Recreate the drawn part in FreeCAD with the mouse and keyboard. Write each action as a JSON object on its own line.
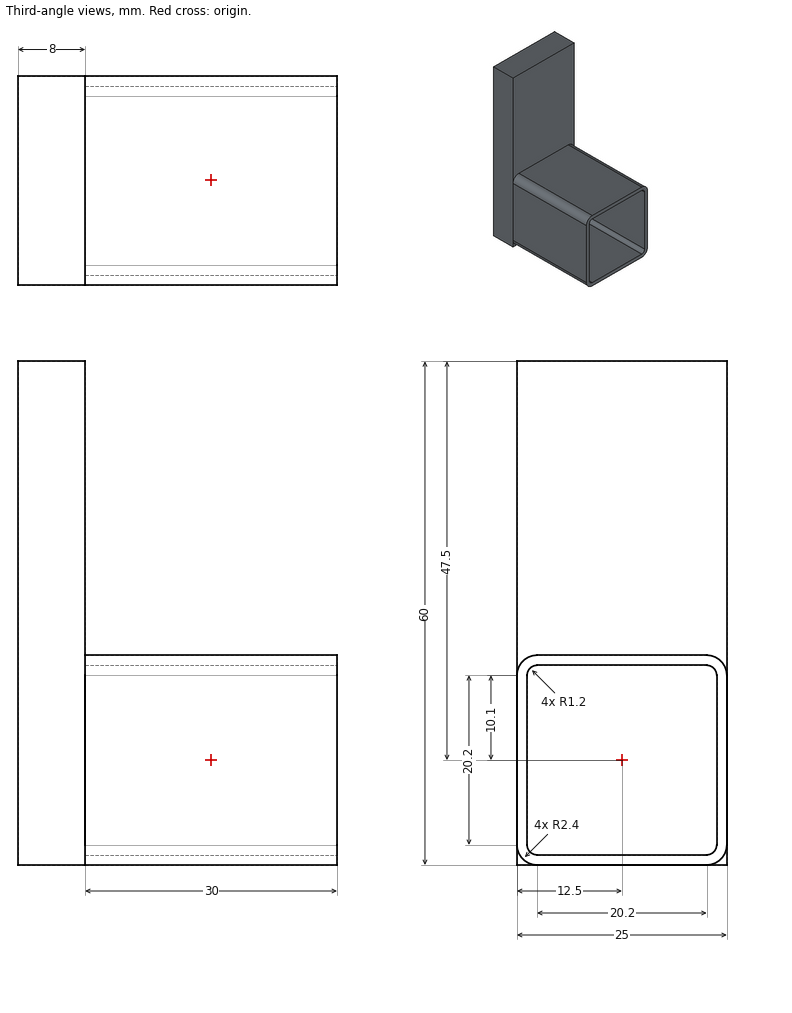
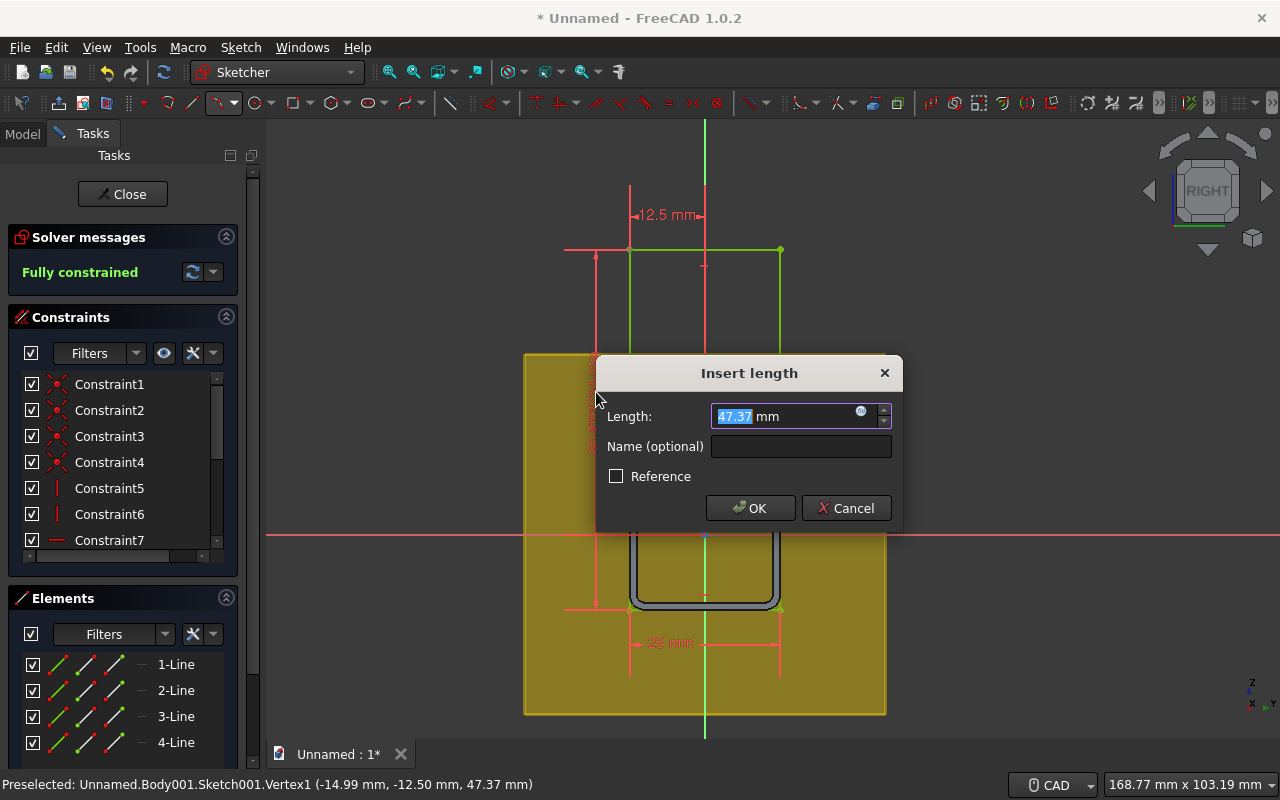
{"action": "type", "text": "47.5"}
{"action": "key", "text": "Return"}
{"action": "key", "text": "Escape"}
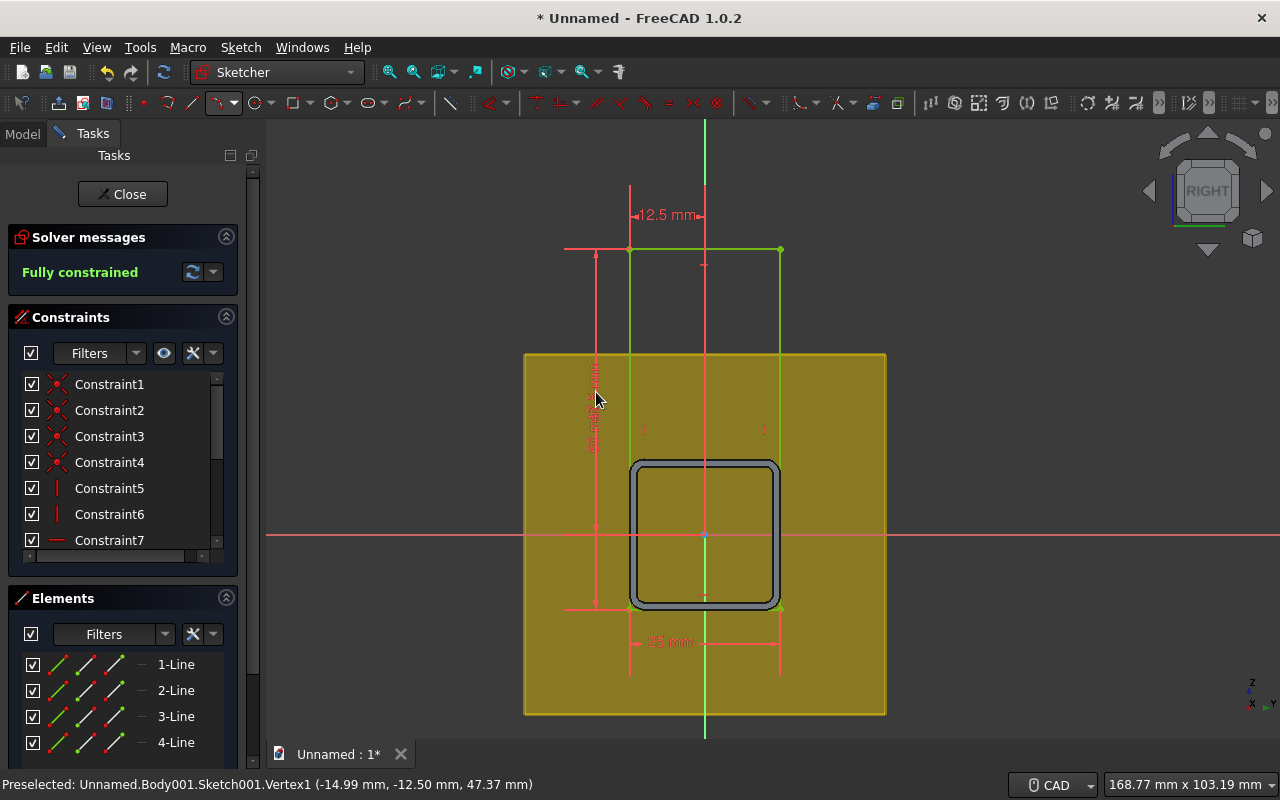
{"action": "left_click", "coordinate": [123, 194]}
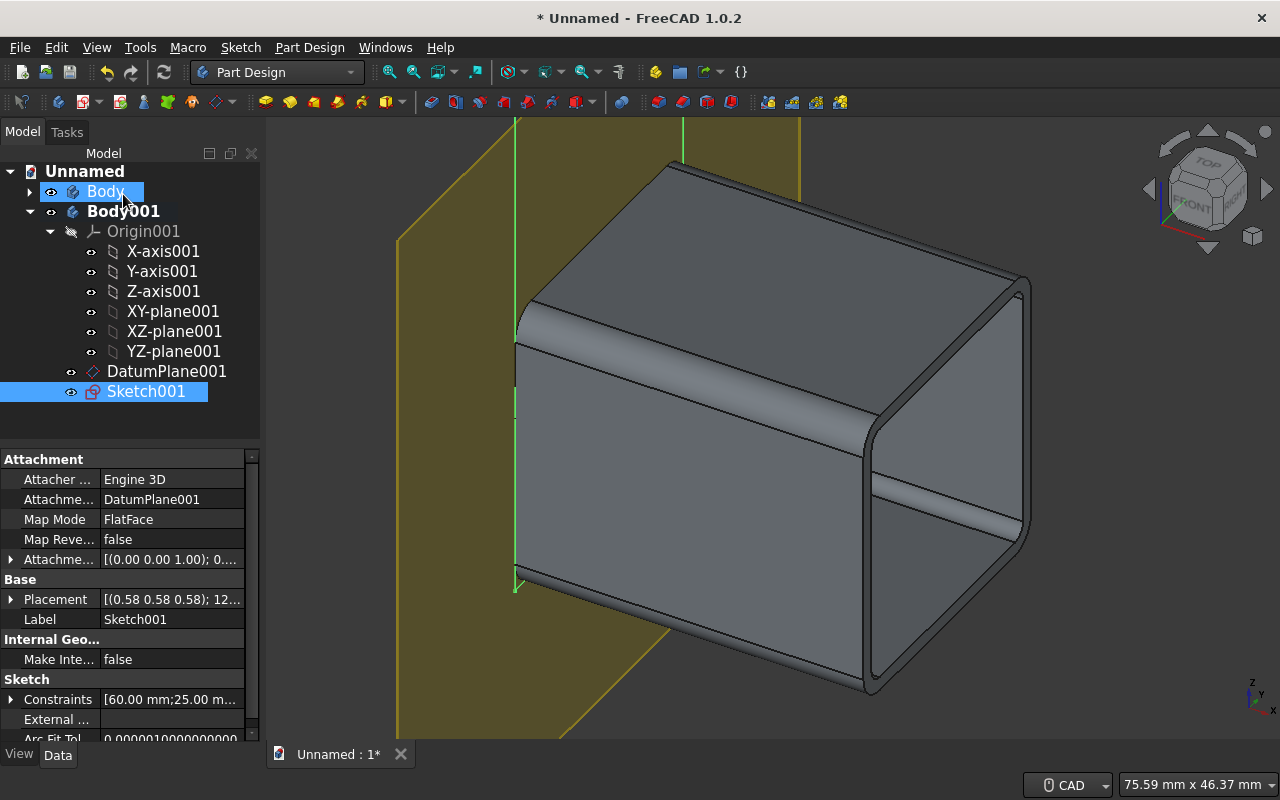
{"action": "left_click", "coordinate": [266, 102]}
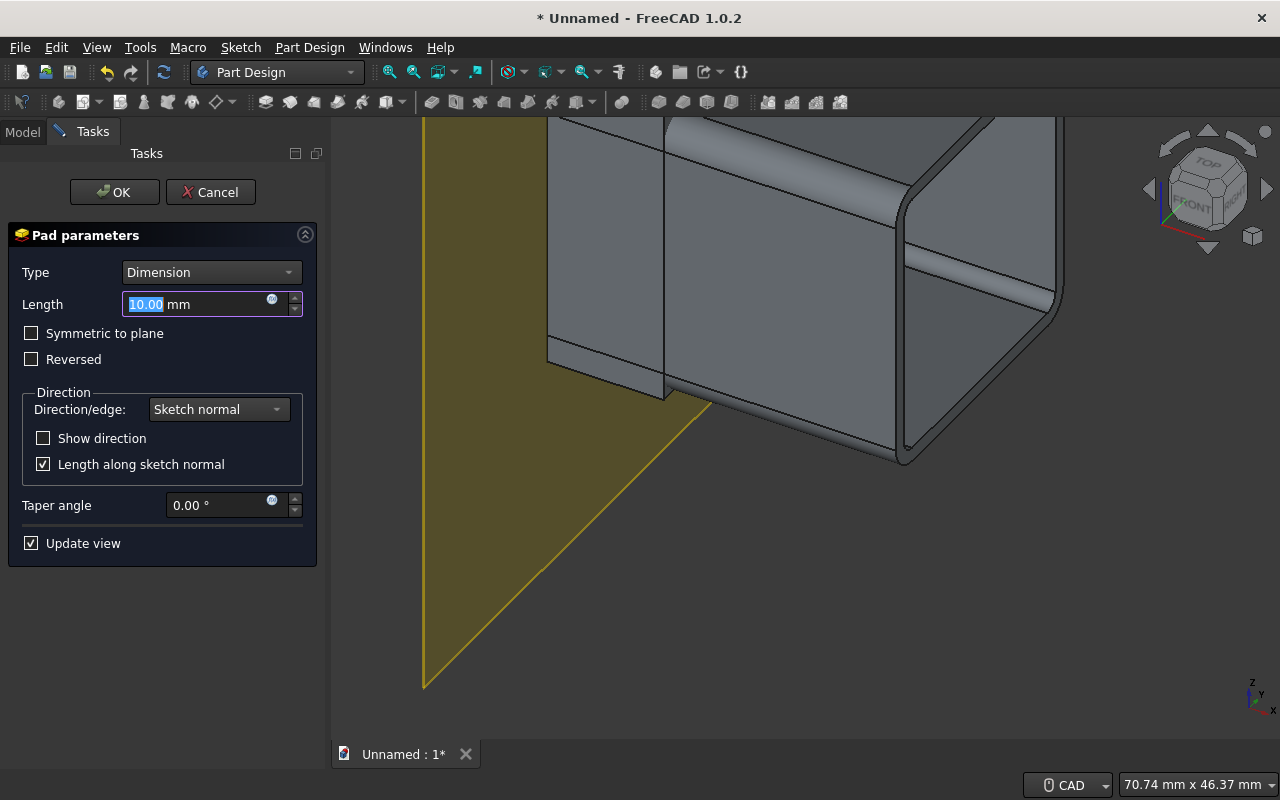
{"action": "type", "text": "8"}
{"action": "key", "text": "Tab"}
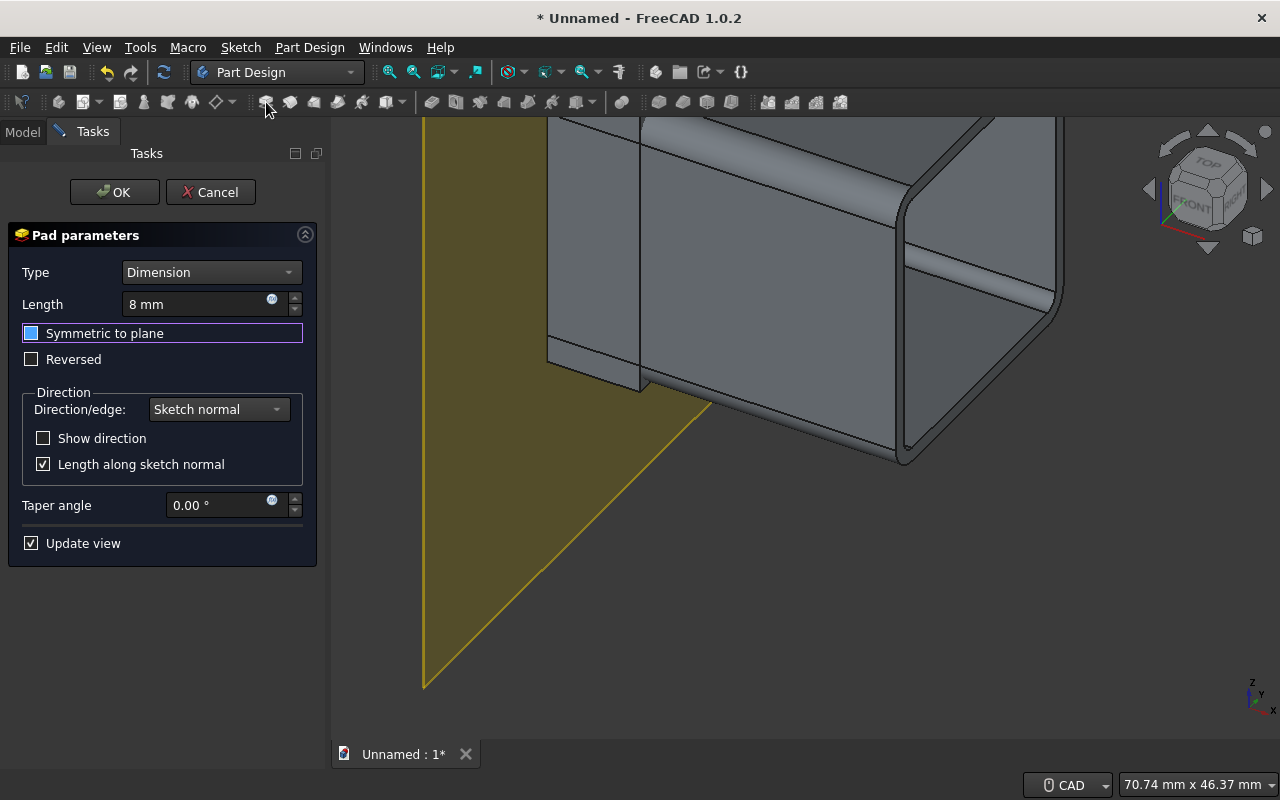
{"action": "left_click", "coordinate": [30, 359]}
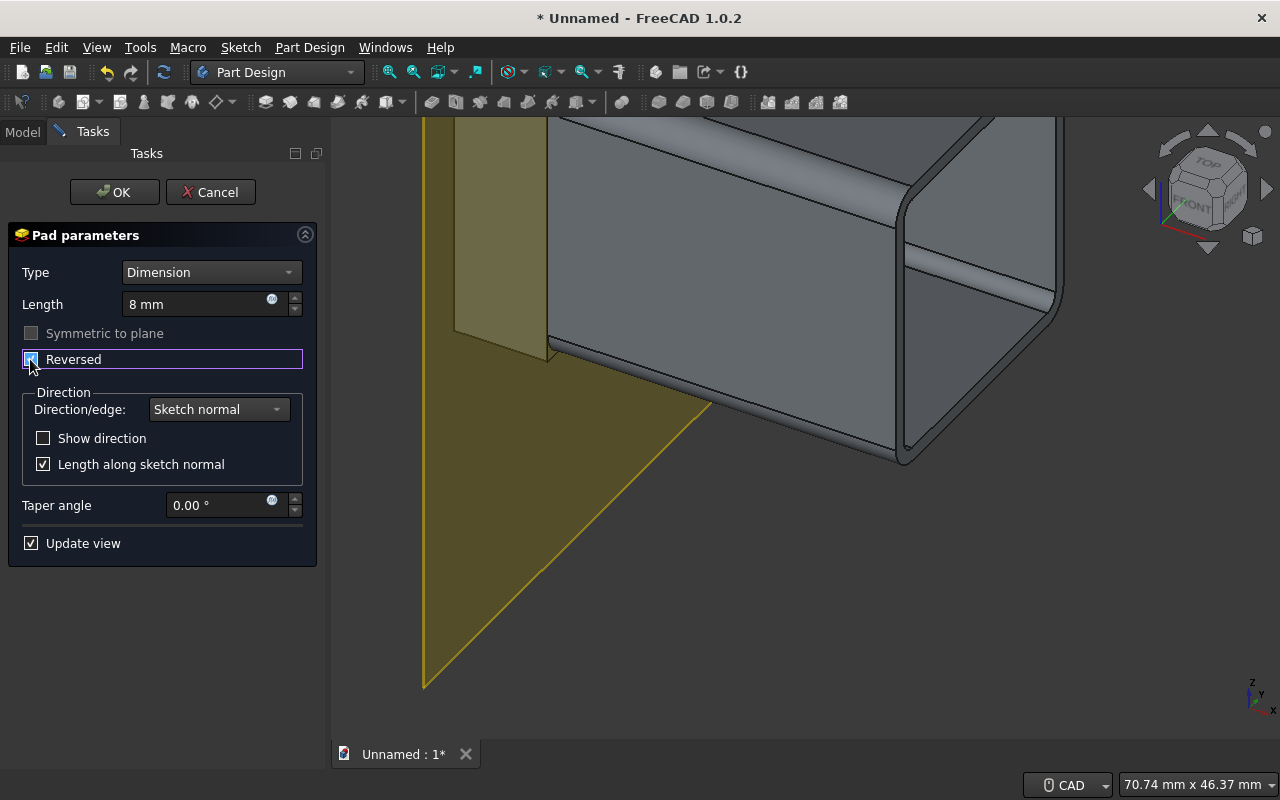
{"action": "left_click", "coordinate": [115, 192]}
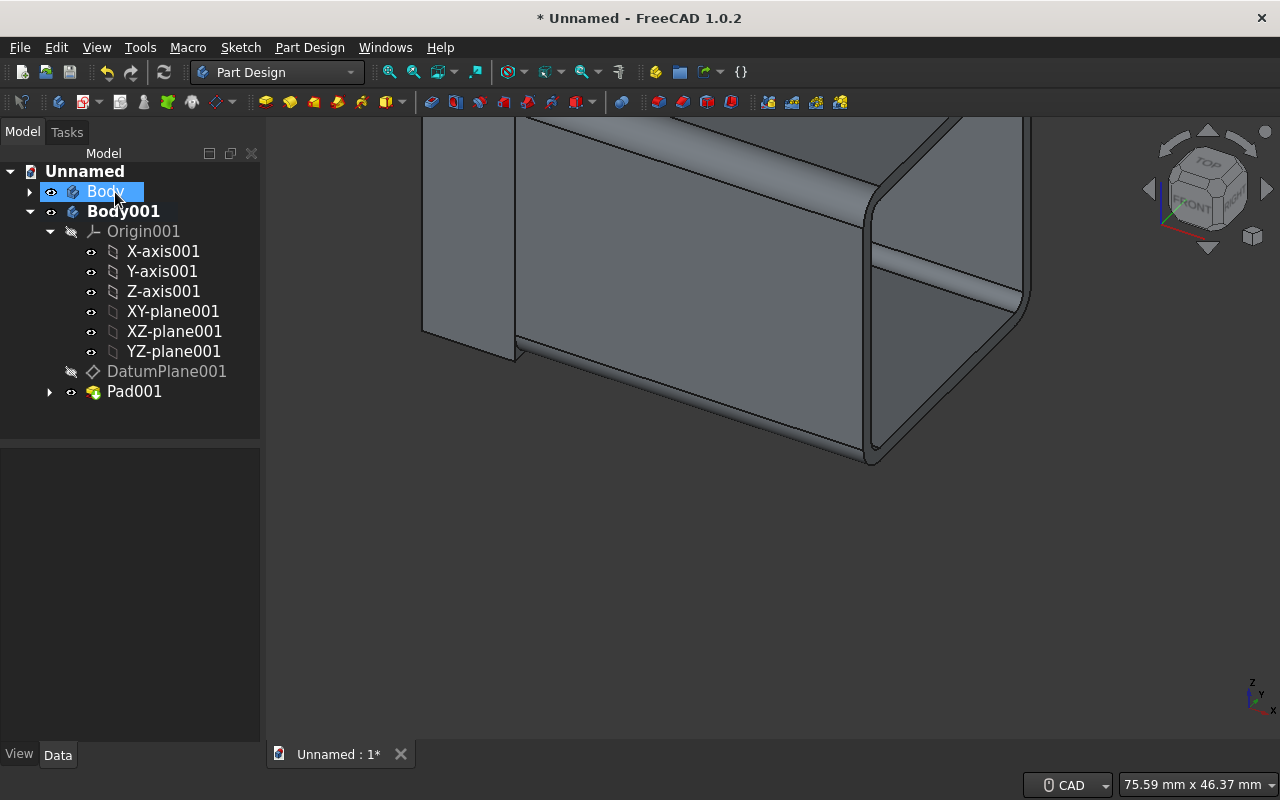
{"action": "key", "text": "0"}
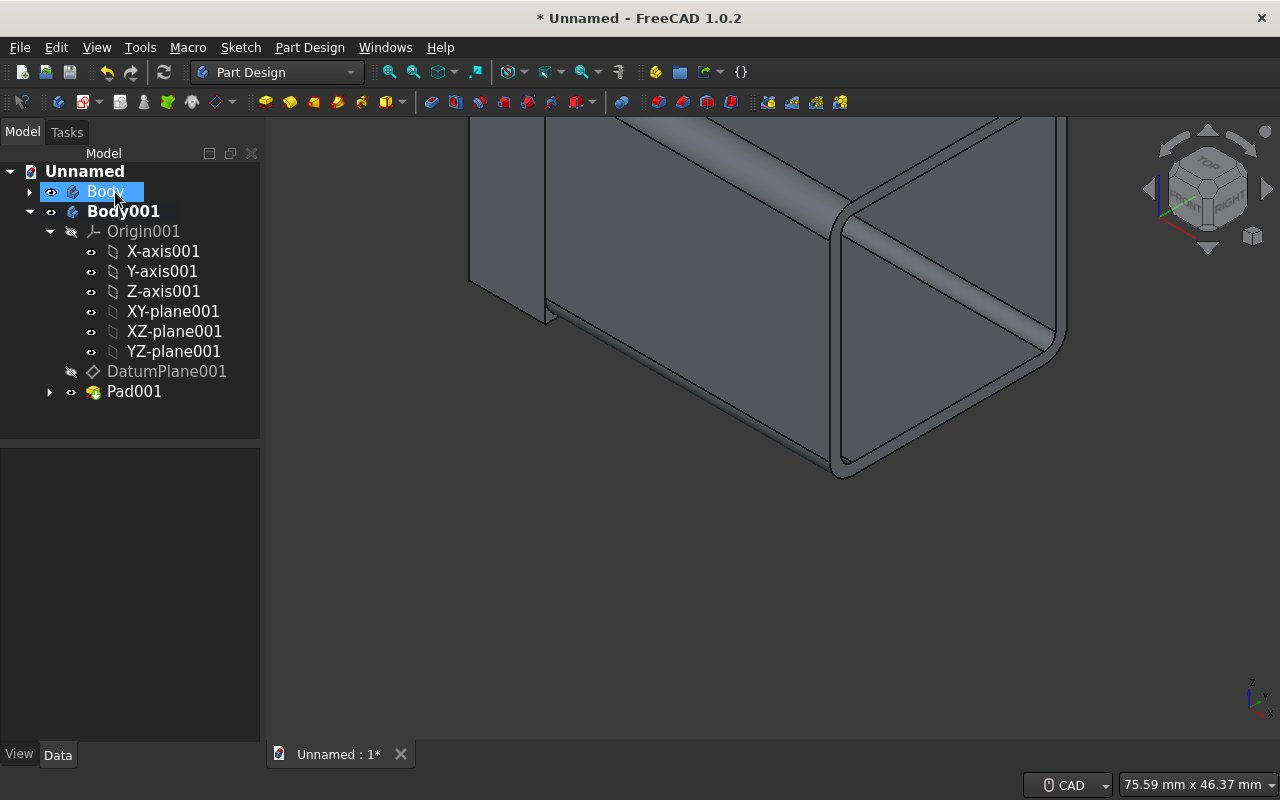
{"action": "key", "text": "v f"}